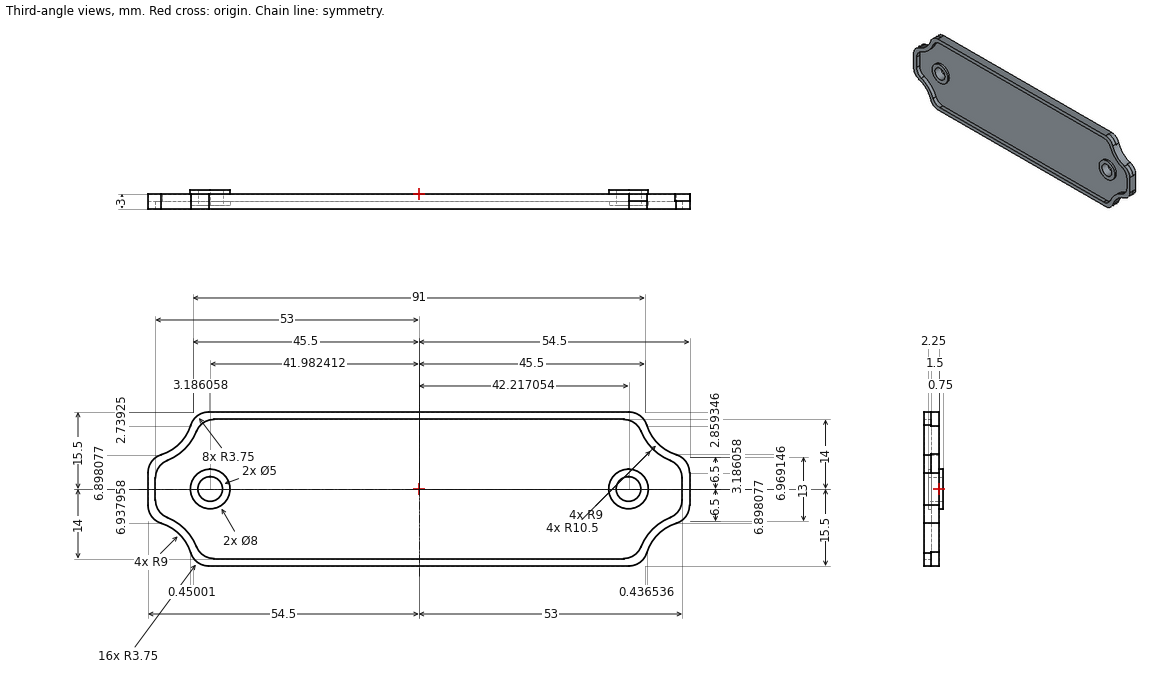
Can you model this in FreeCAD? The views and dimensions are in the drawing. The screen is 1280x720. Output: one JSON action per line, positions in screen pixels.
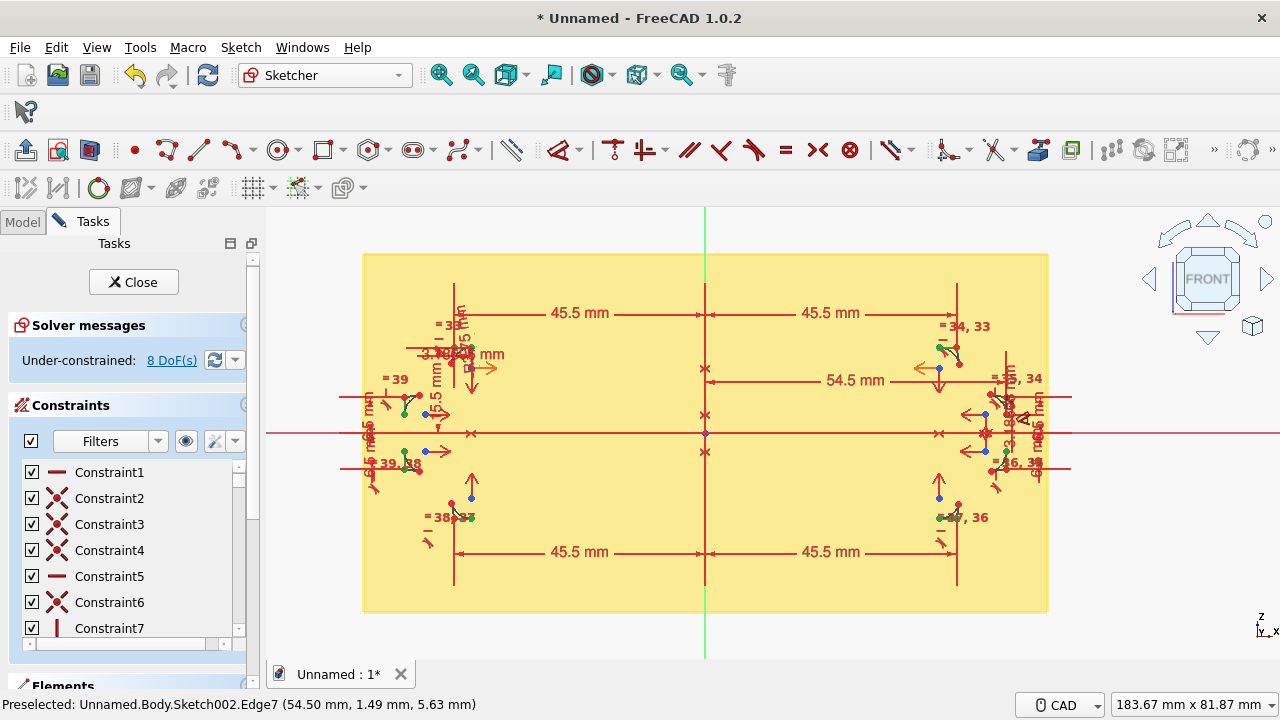
{"action": "scroll", "coordinate": [454, 352], "scroll_direction": "up", "scroll_amount": 7}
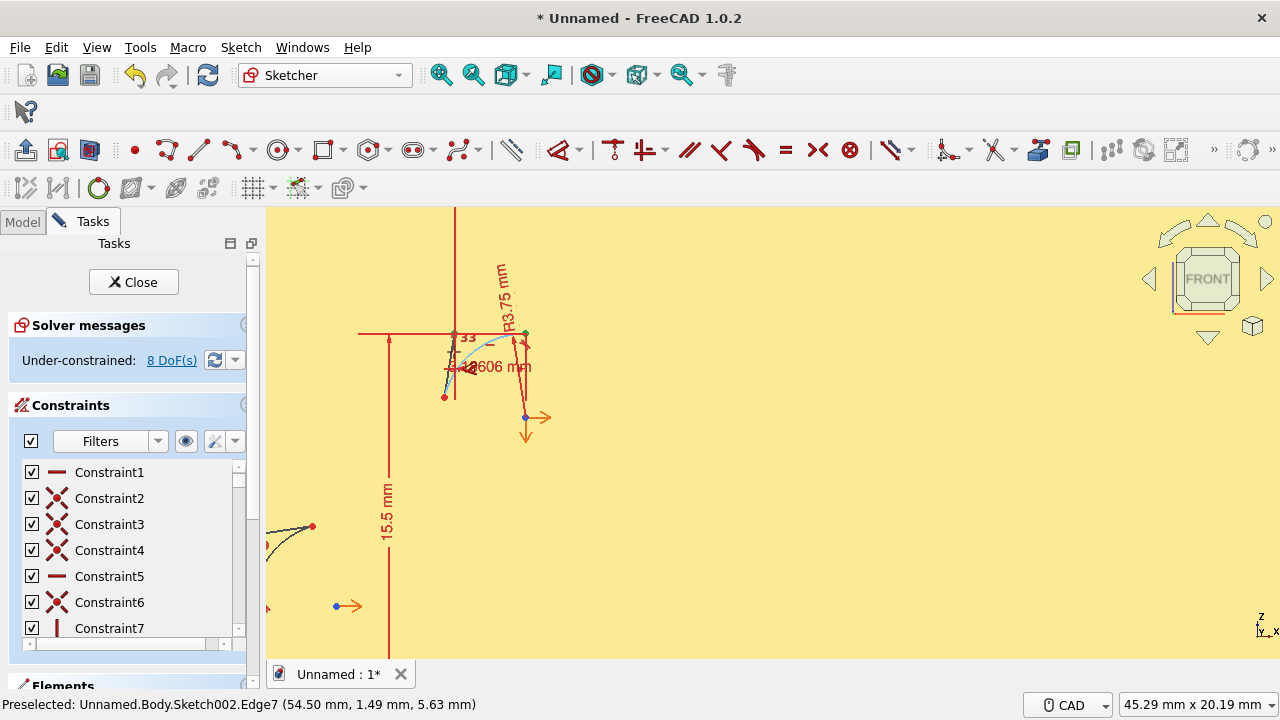
{"action": "left_click", "coordinate": [451, 353]}
{"action": "left_click", "coordinate": [410, 365]}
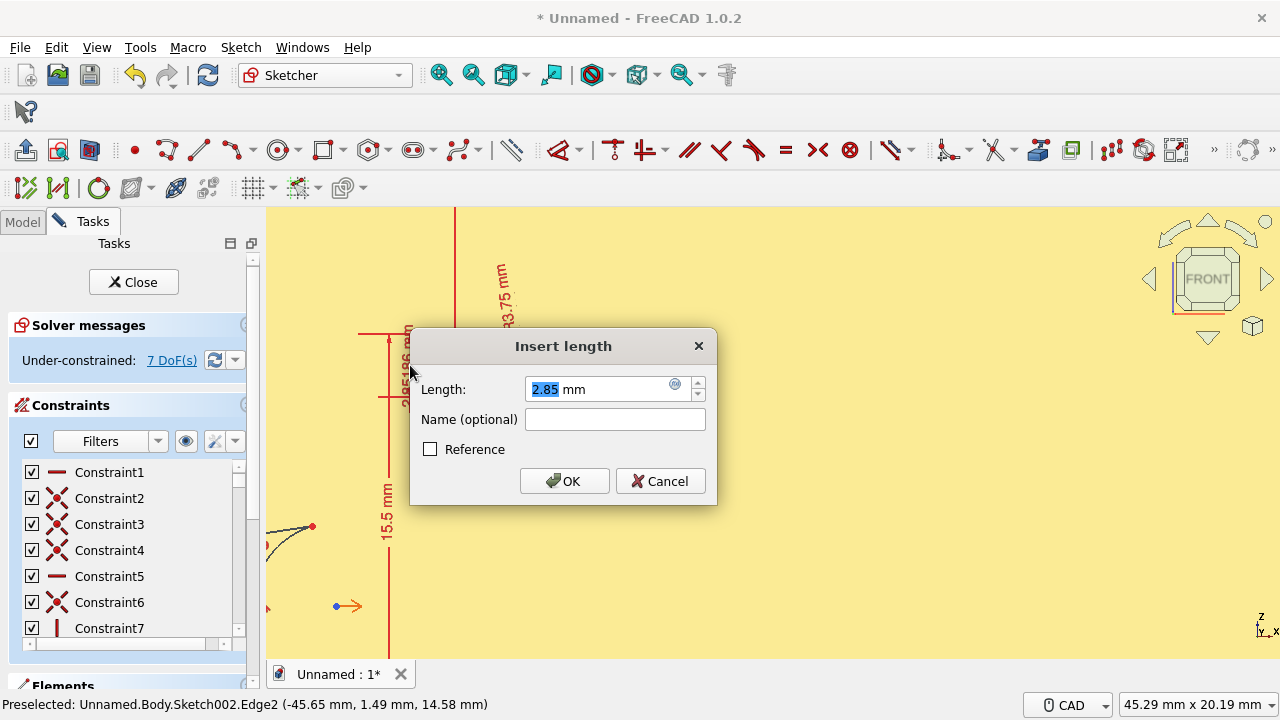
{"action": "type", "text": "2.73925"}
{"action": "key", "text": "Return"}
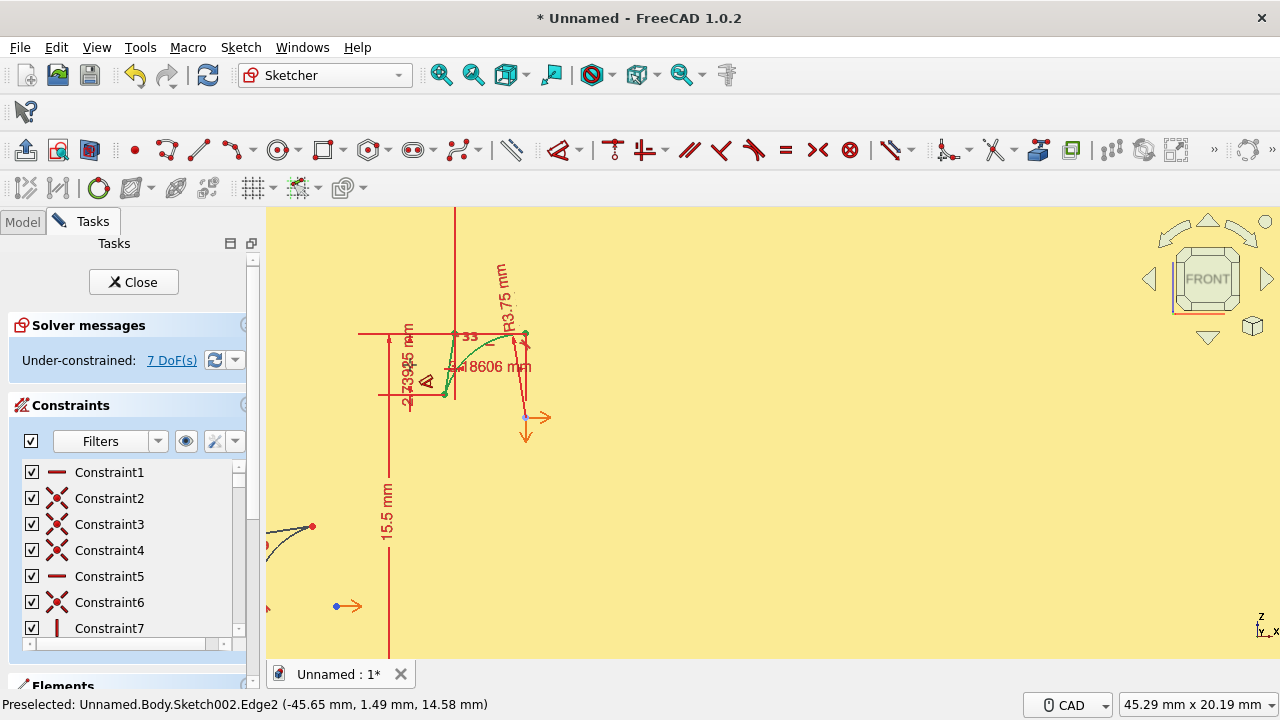
{"action": "scroll", "coordinate": [453, 352], "scroll_direction": "down", "scroll_amount": 7}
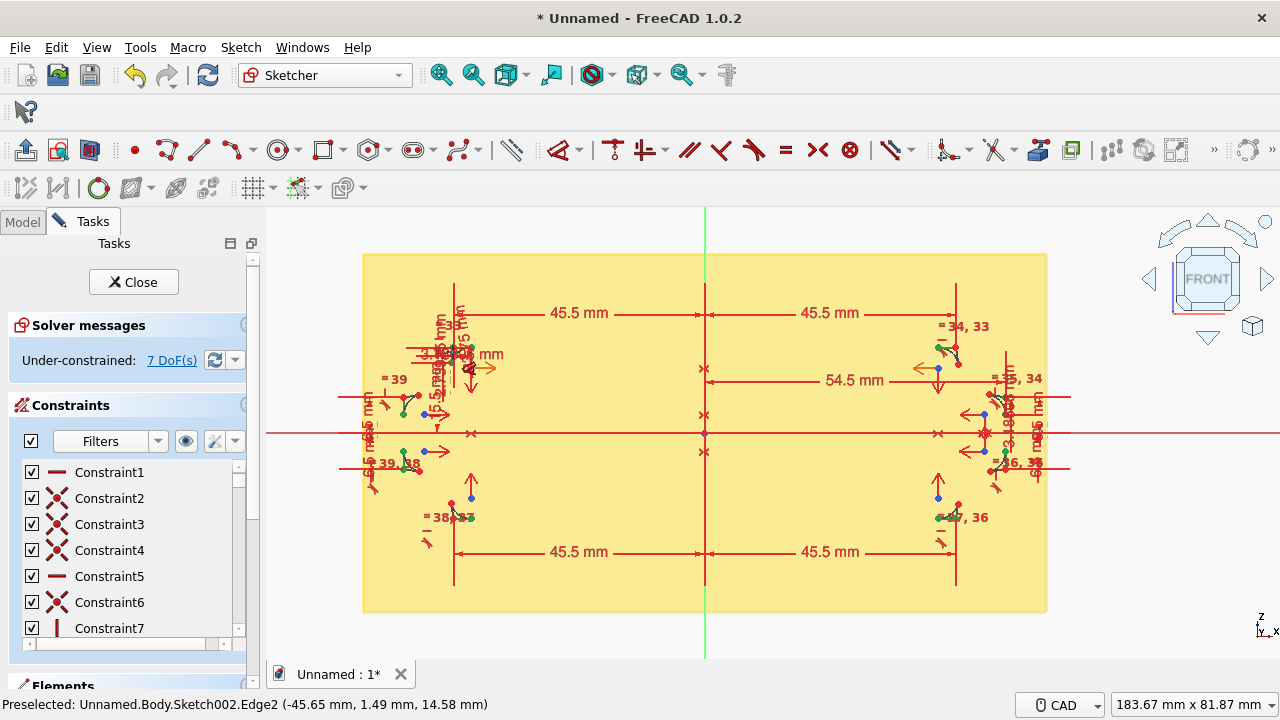
{"action": "scroll", "coordinate": [453, 514], "scroll_direction": "up", "scroll_amount": 14}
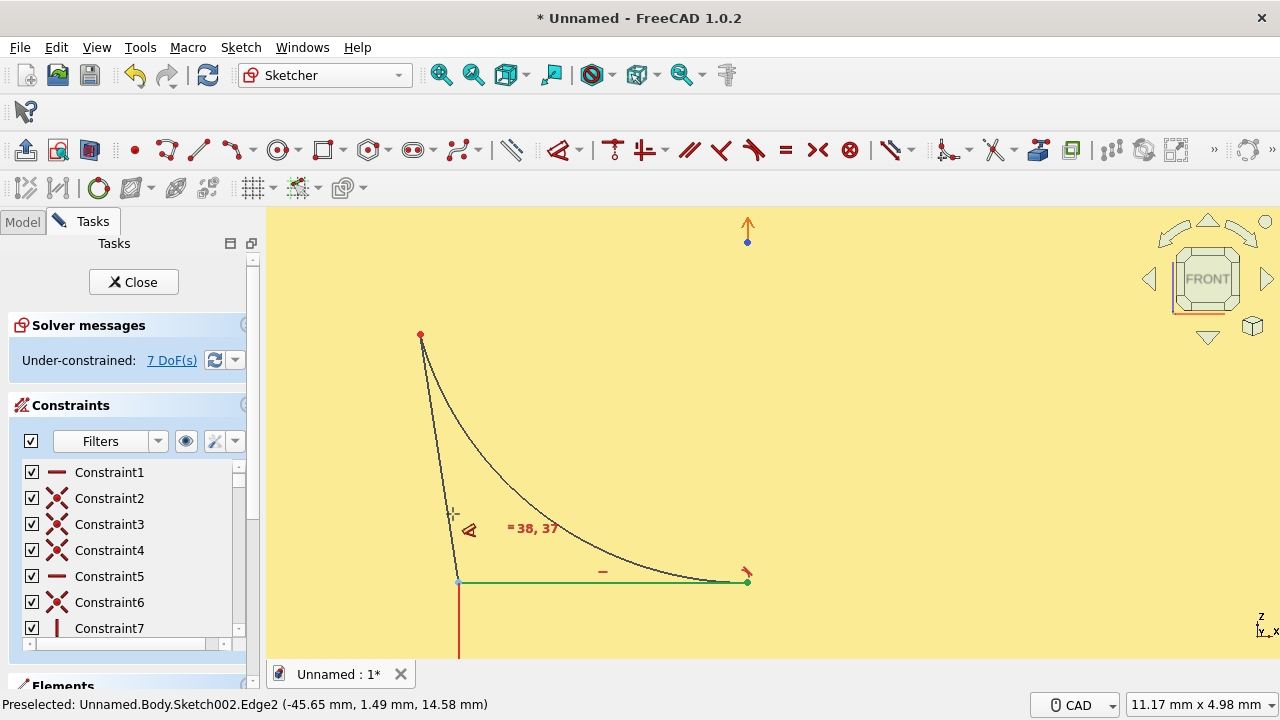
{"action": "left_click", "coordinate": [447, 508]}
{"action": "left_click", "coordinate": [439, 617]}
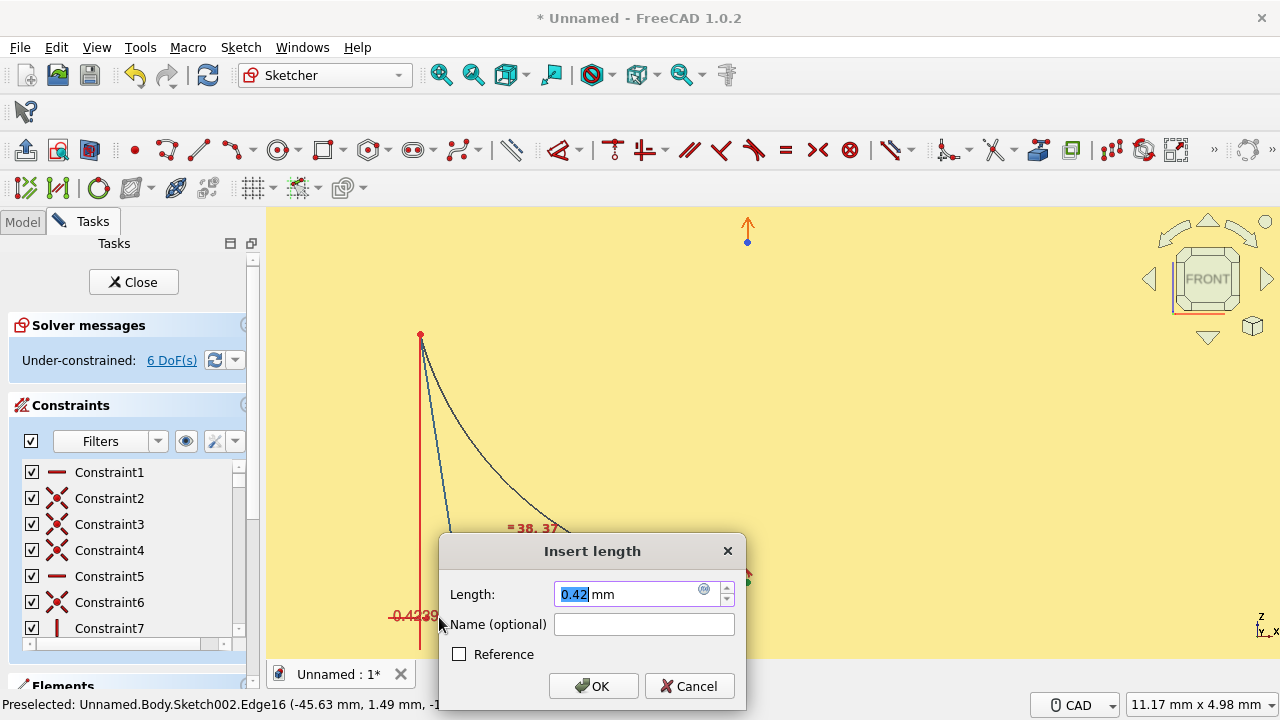
{"action": "type", "text": "0.45001"}
{"action": "key", "text": "Return"}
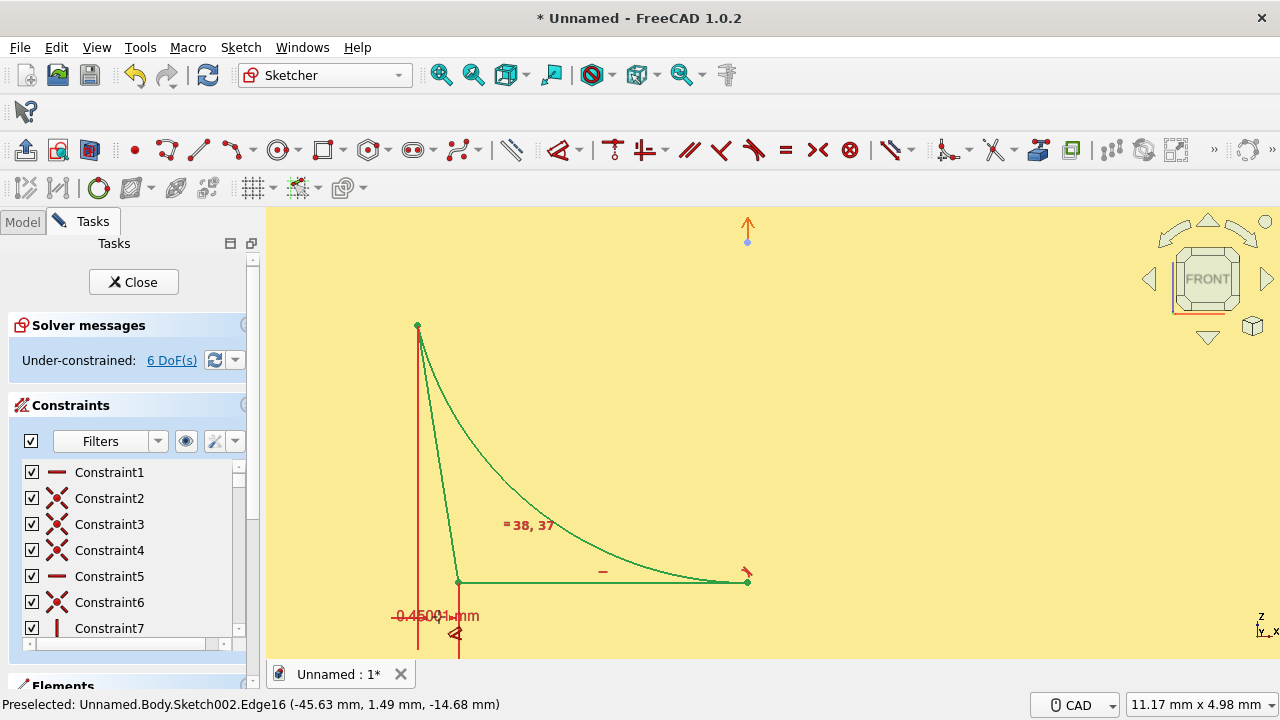
{"action": "scroll", "coordinate": [453, 514], "scroll_direction": "down", "scroll_amount": 14}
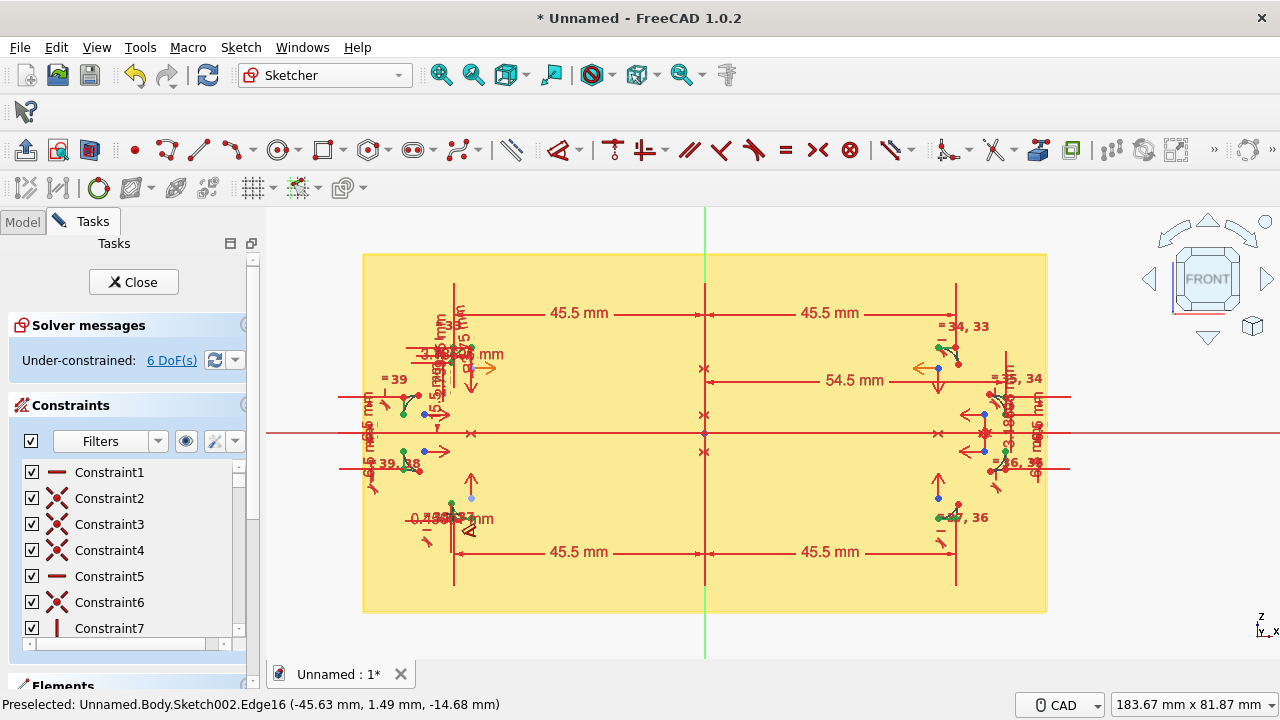
{"action": "left_click", "coordinate": [989, 395]}
{"action": "left_click", "coordinate": [671, 414]}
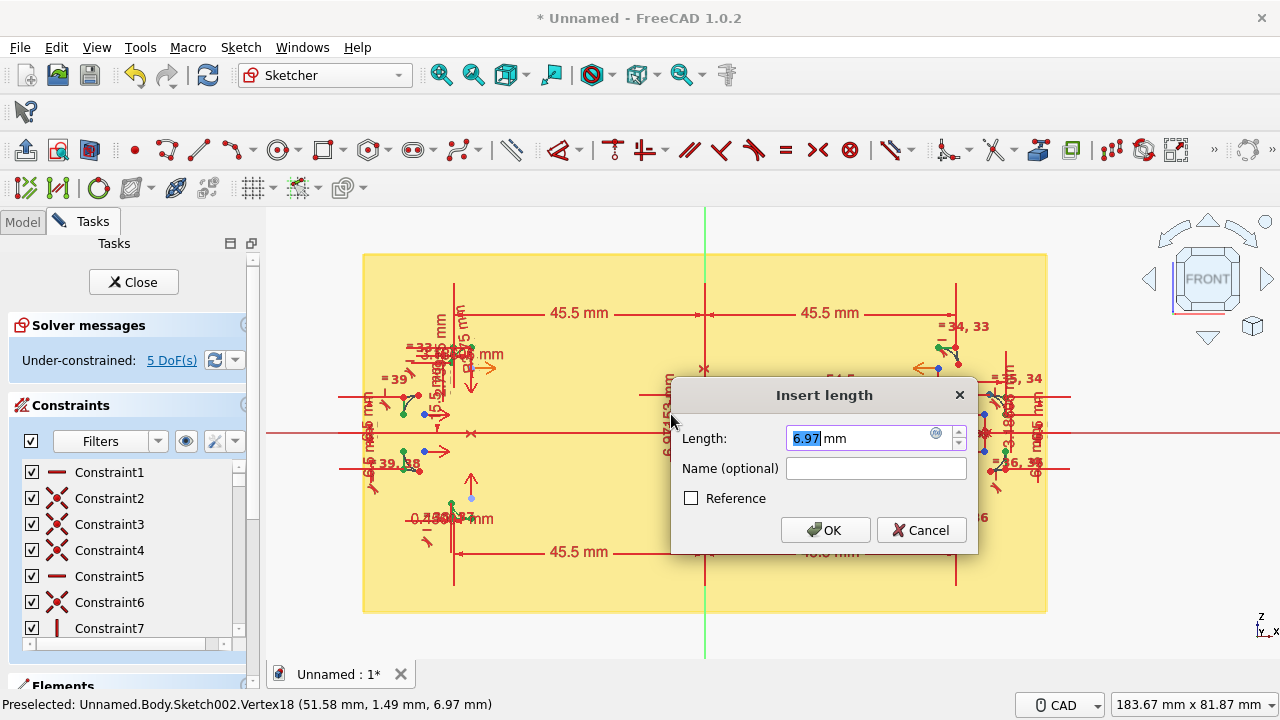
{"action": "type", "text": "6.969146"}
{"action": "key", "text": "Return"}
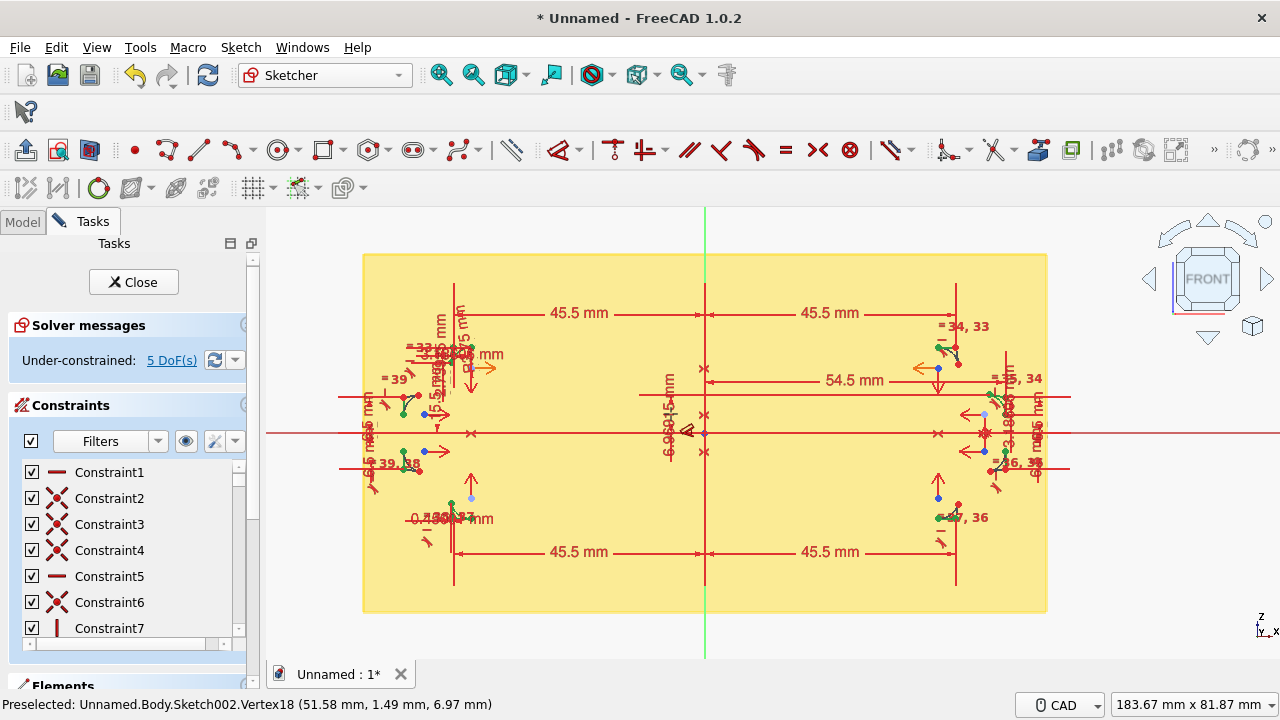
{"action": "left_click", "coordinate": [991, 471]}
{"action": "left_click", "coordinate": [671, 452]}